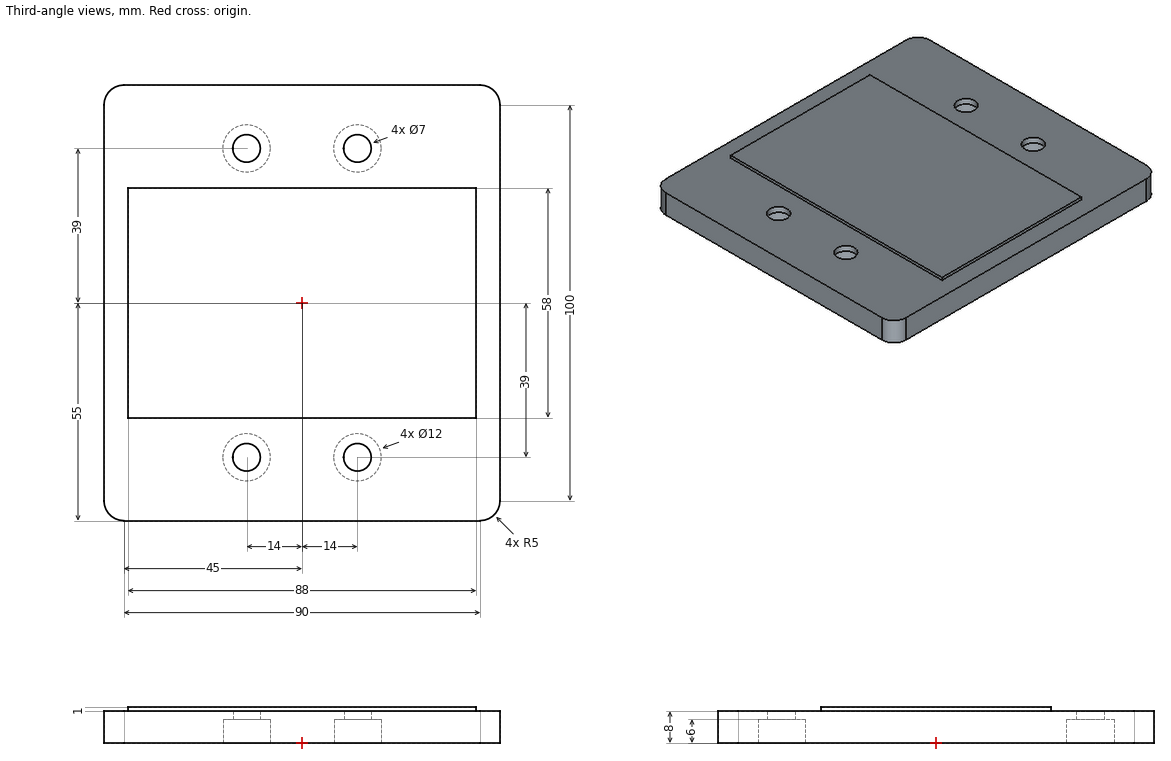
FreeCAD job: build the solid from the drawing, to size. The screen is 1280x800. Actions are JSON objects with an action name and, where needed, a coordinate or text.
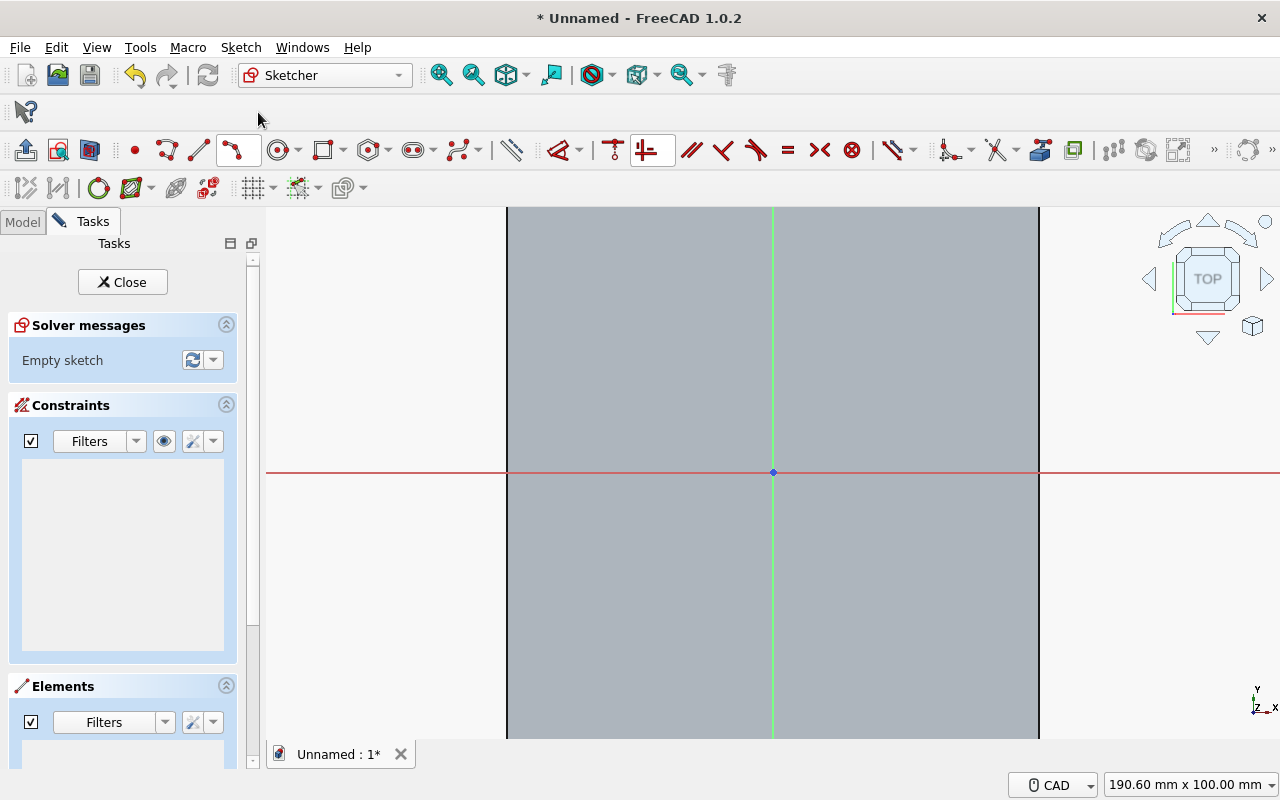
{"action": "key", "text": "g v"}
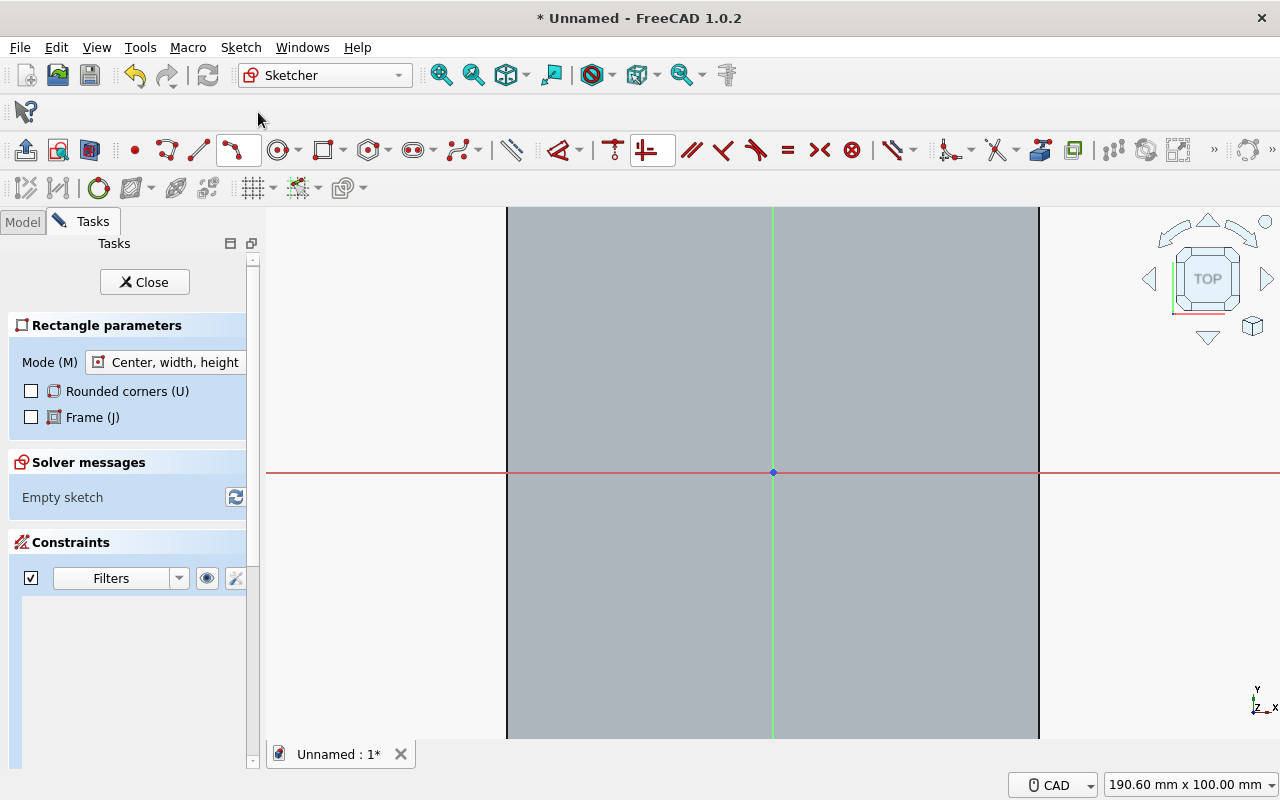
{"action": "left_click", "coordinate": [773, 473]}
{"action": "mouse_move", "coordinate": [1007, 319]}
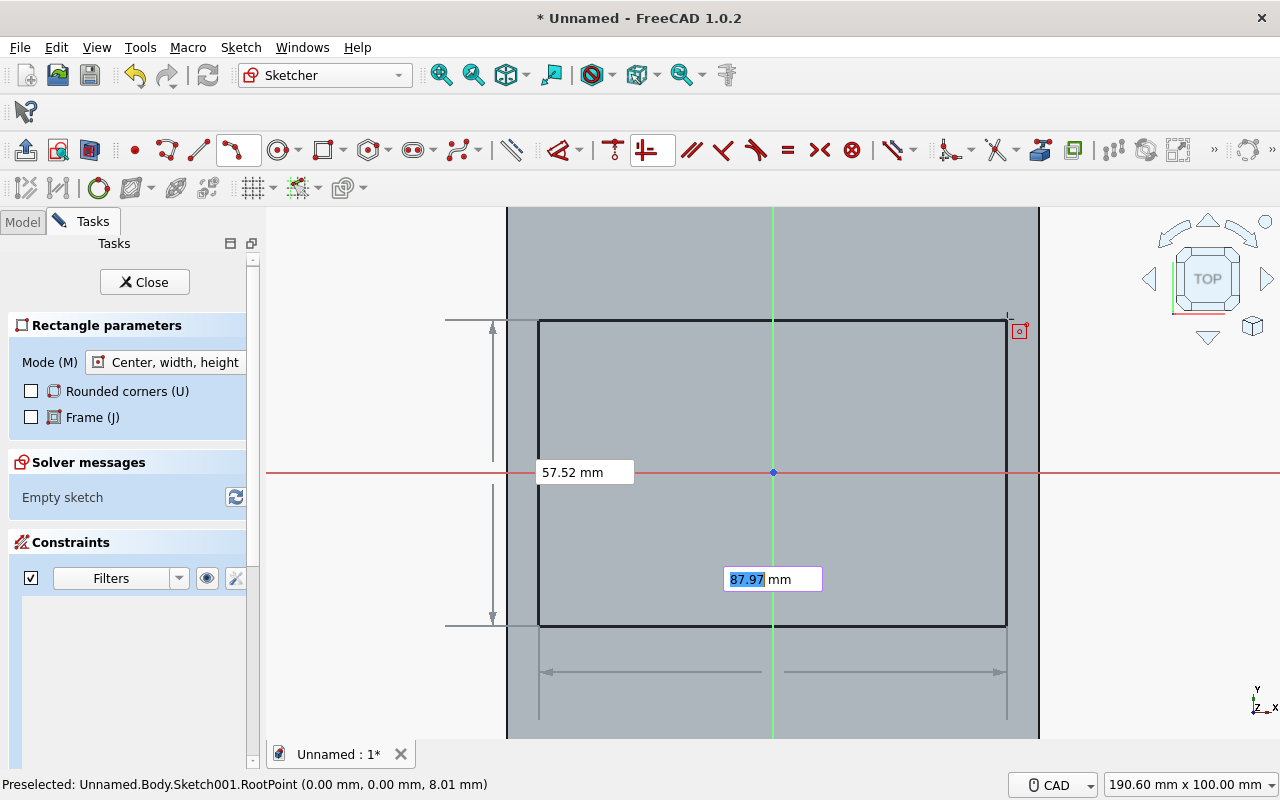
{"action": "type", "text": "88"}
{"action": "key", "text": "Tab"}
{"action": "type", "text": "58"}
{"action": "key", "text": "Return"}
{"action": "key", "text": "Escape"}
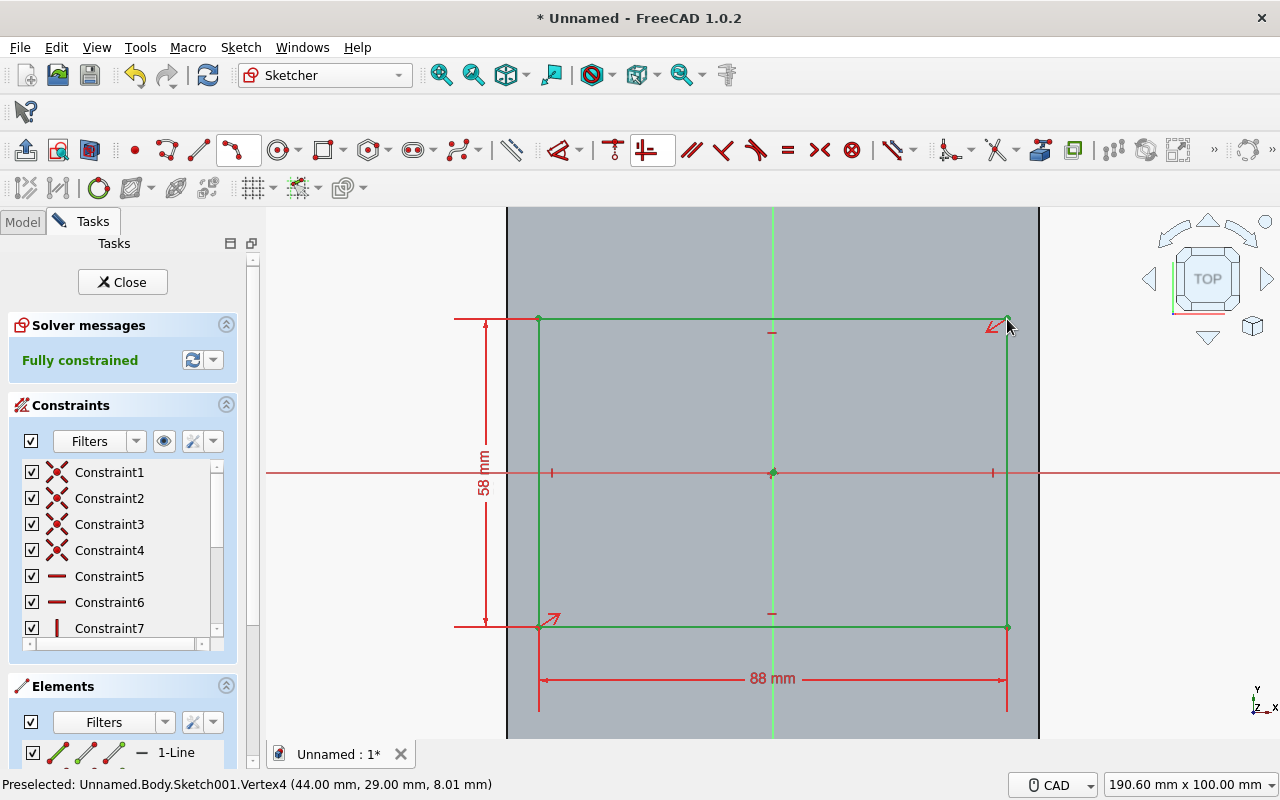
{"action": "left_click", "coordinate": [123, 282]}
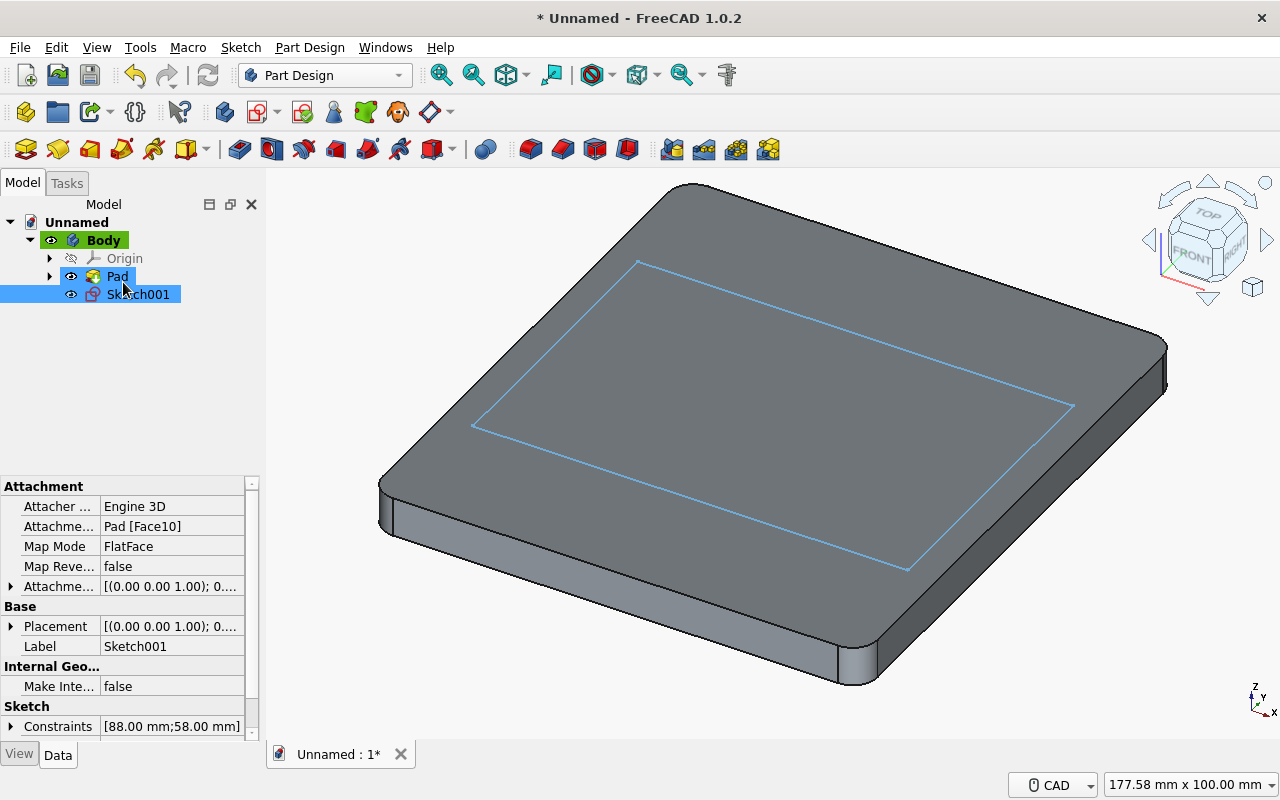
{"action": "left_click", "coordinate": [26, 150]}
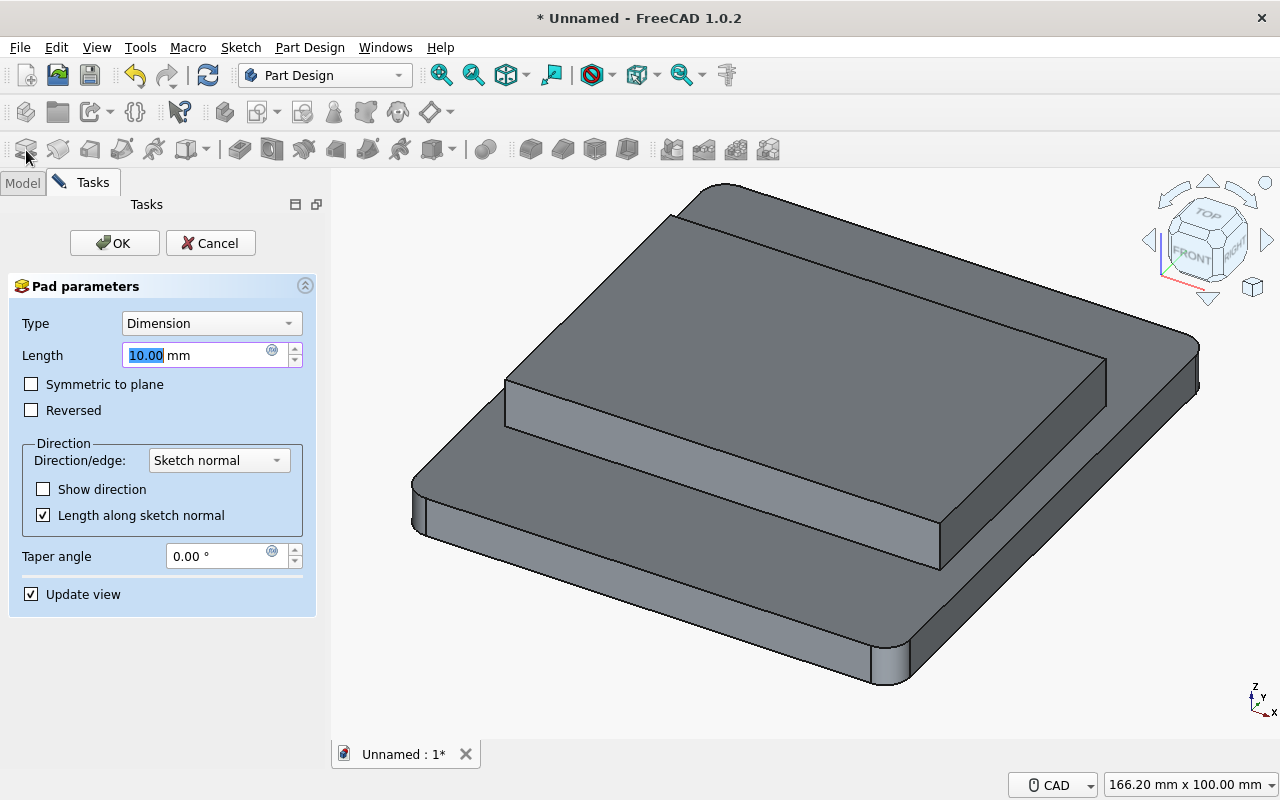
{"action": "type", "text": "1"}
{"action": "key", "text": "Tab"}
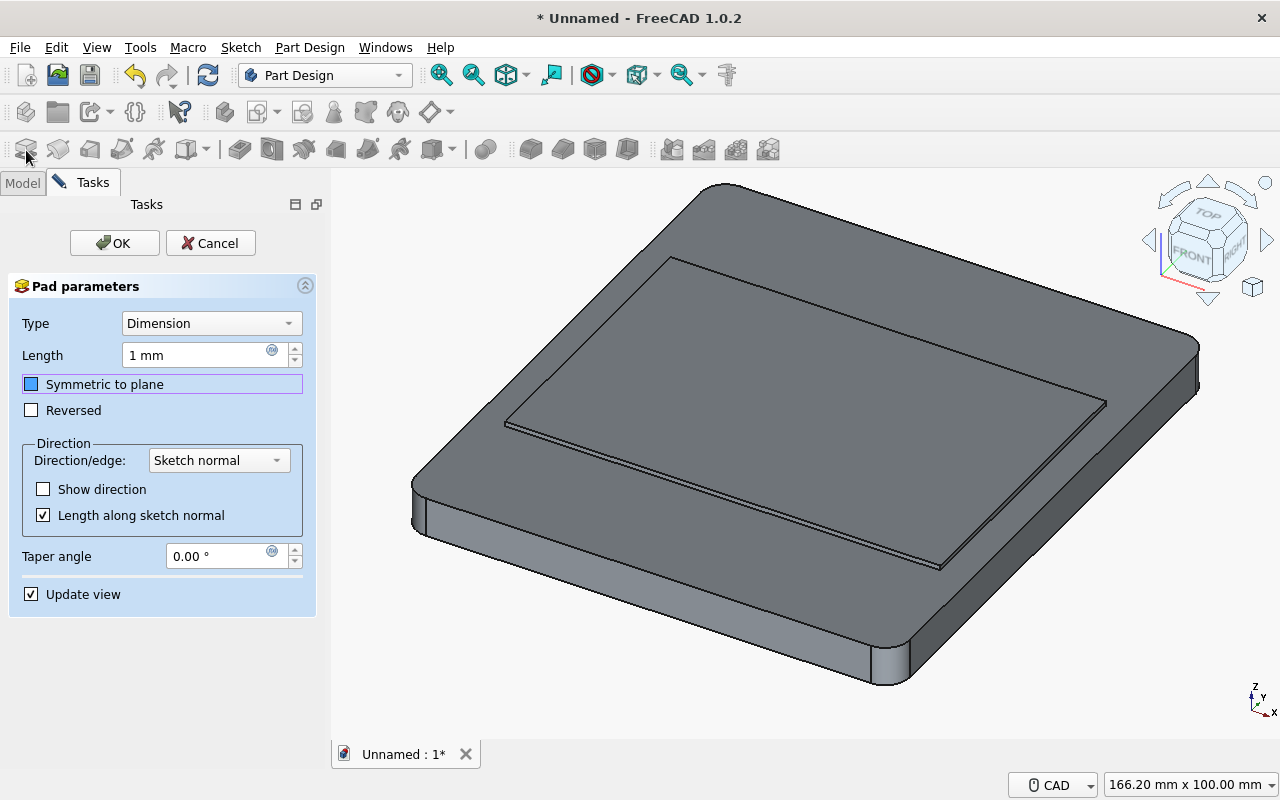
{"action": "left_click", "coordinate": [115, 243]}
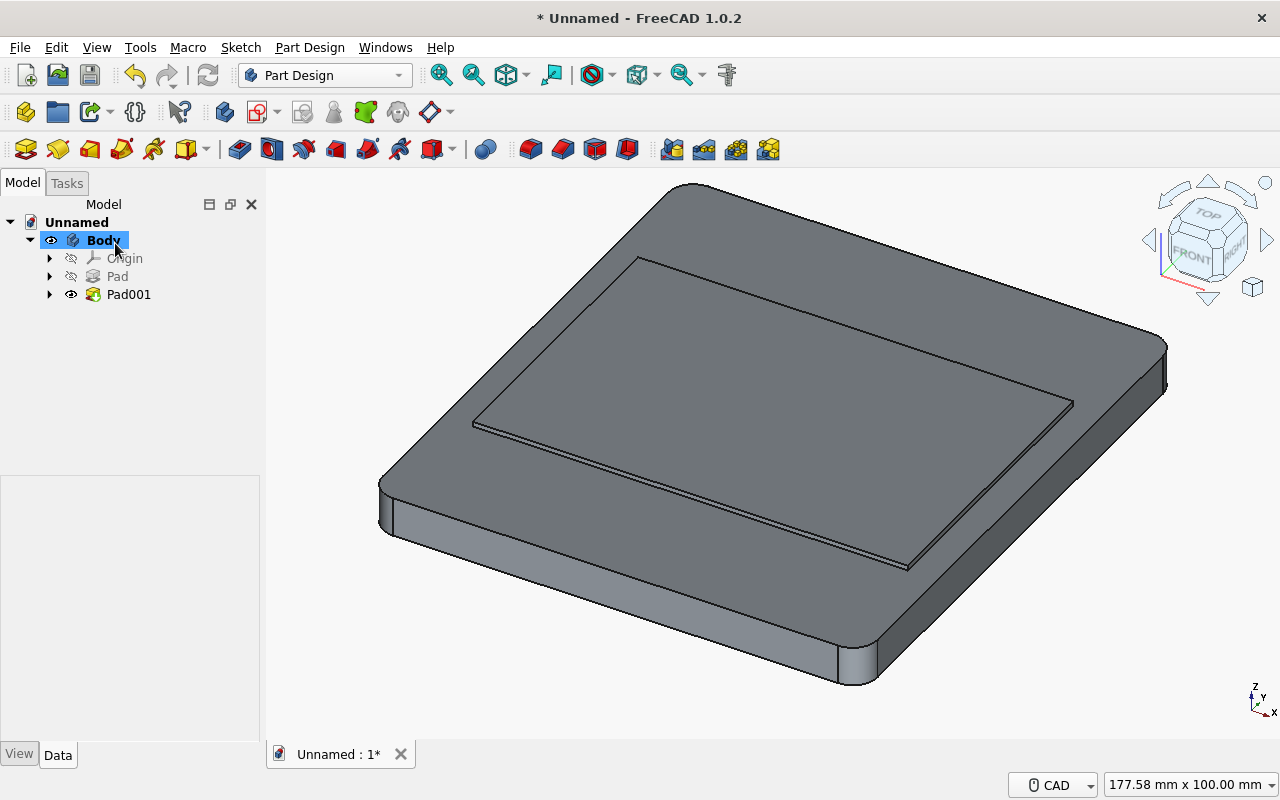
{"action": "left_click", "coordinate": [258, 112]}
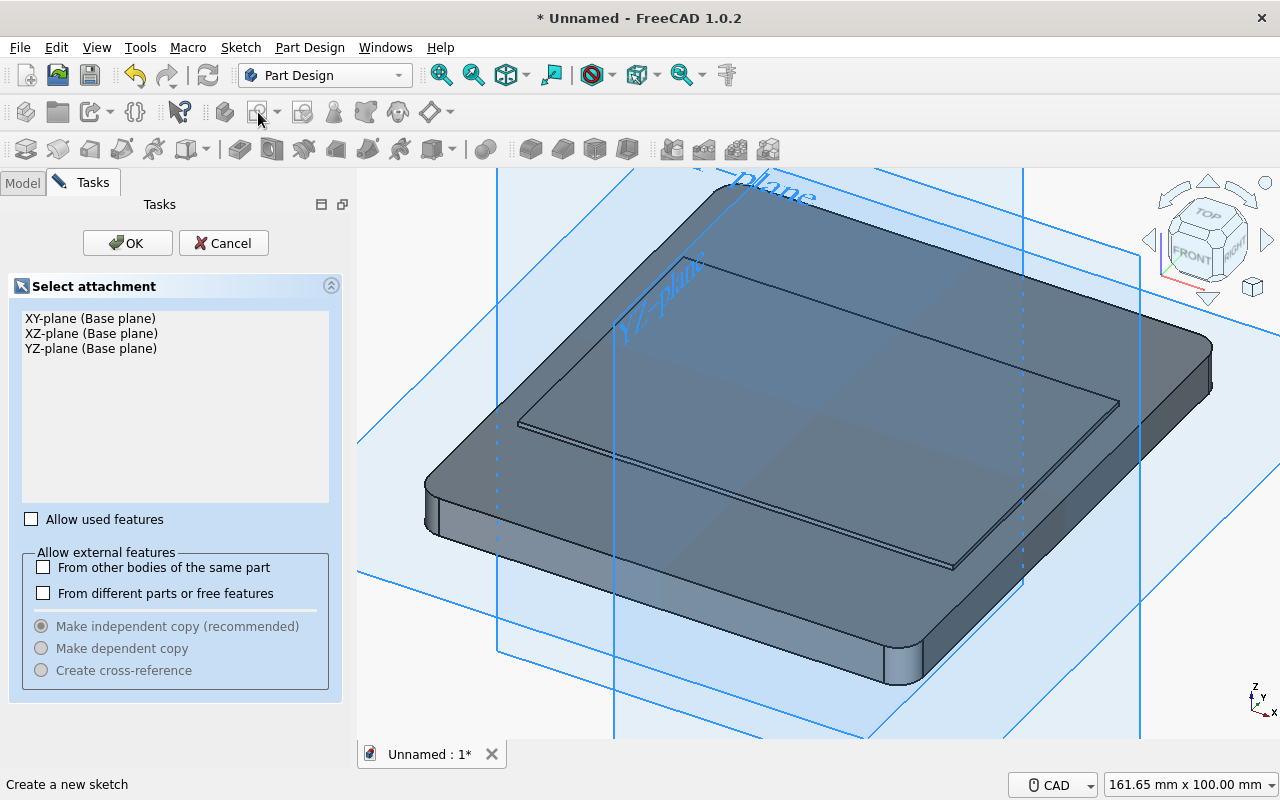
{"action": "left_click", "coordinate": [82, 318]}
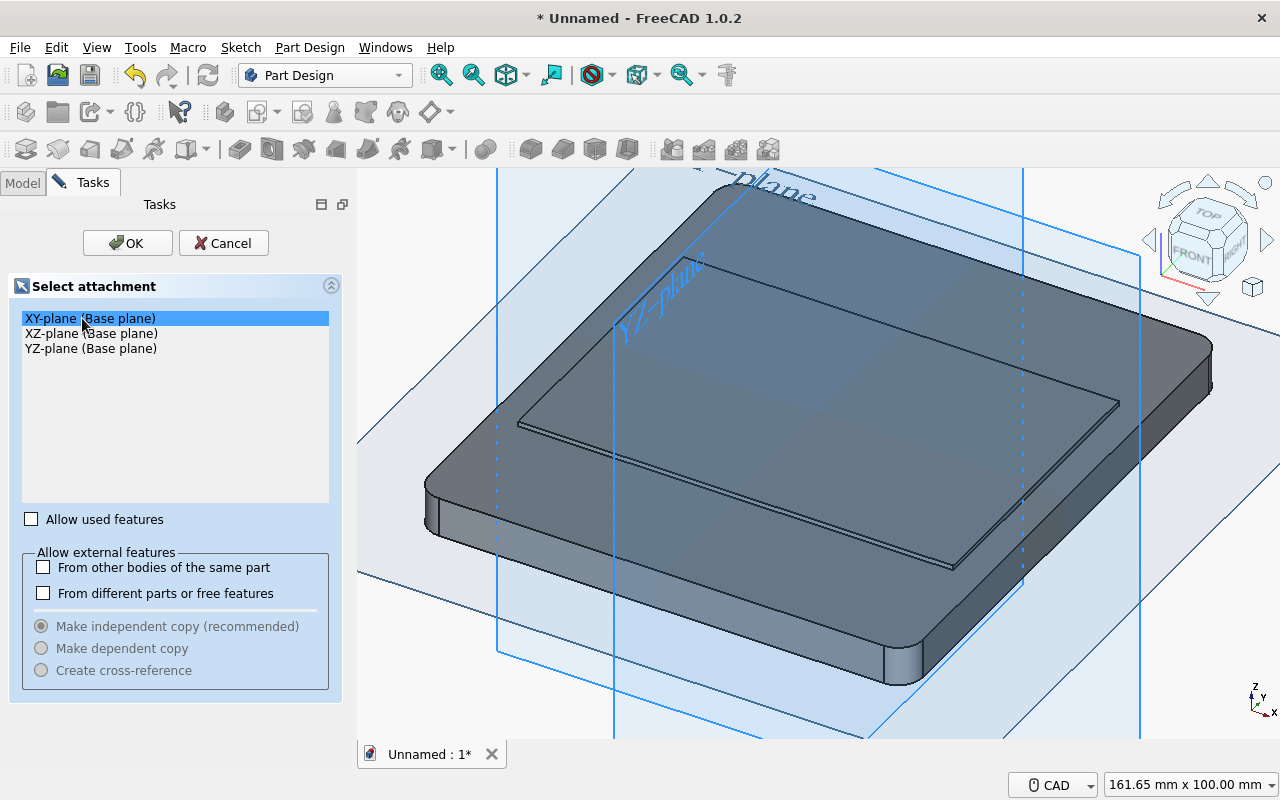
{"action": "left_click", "coordinate": [128, 243]}